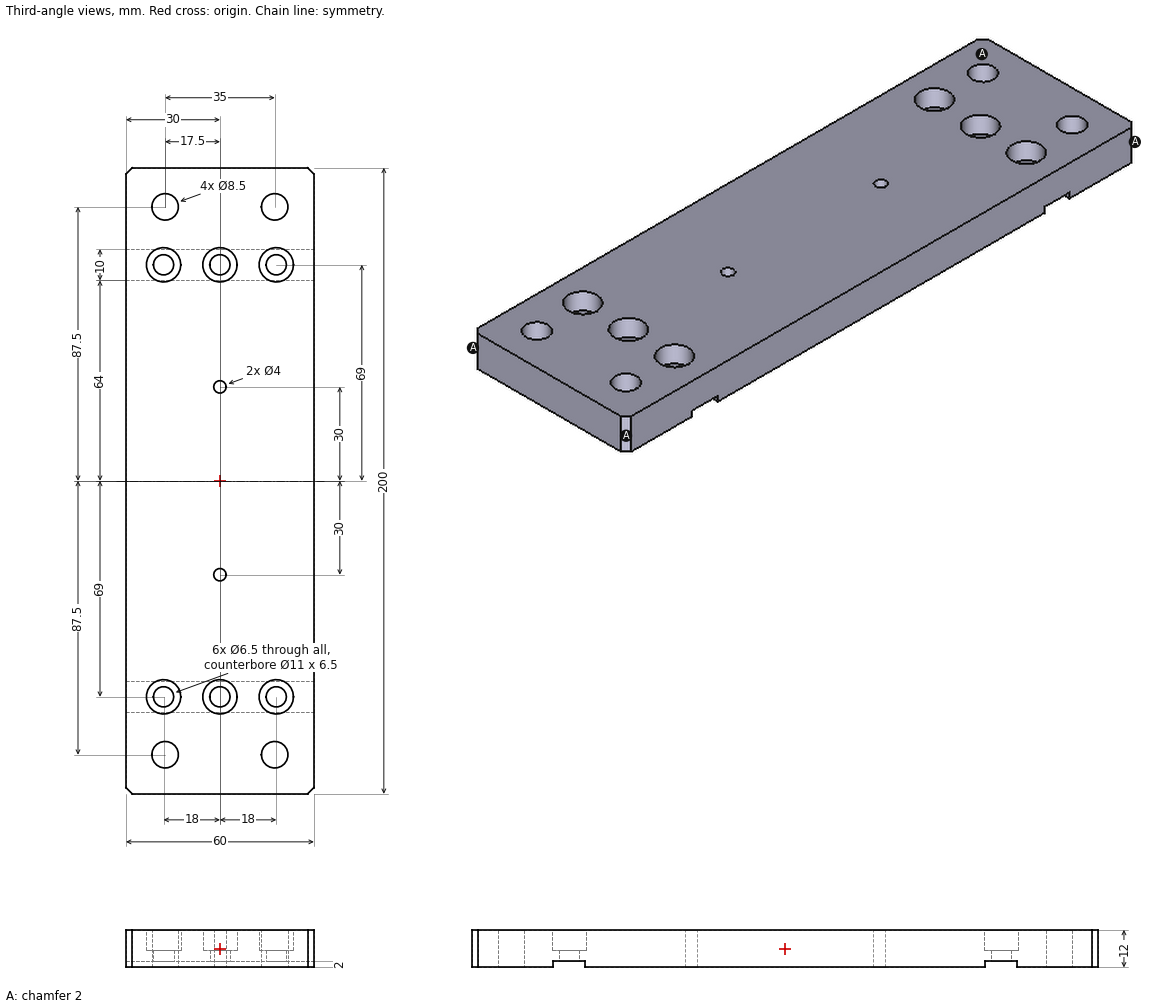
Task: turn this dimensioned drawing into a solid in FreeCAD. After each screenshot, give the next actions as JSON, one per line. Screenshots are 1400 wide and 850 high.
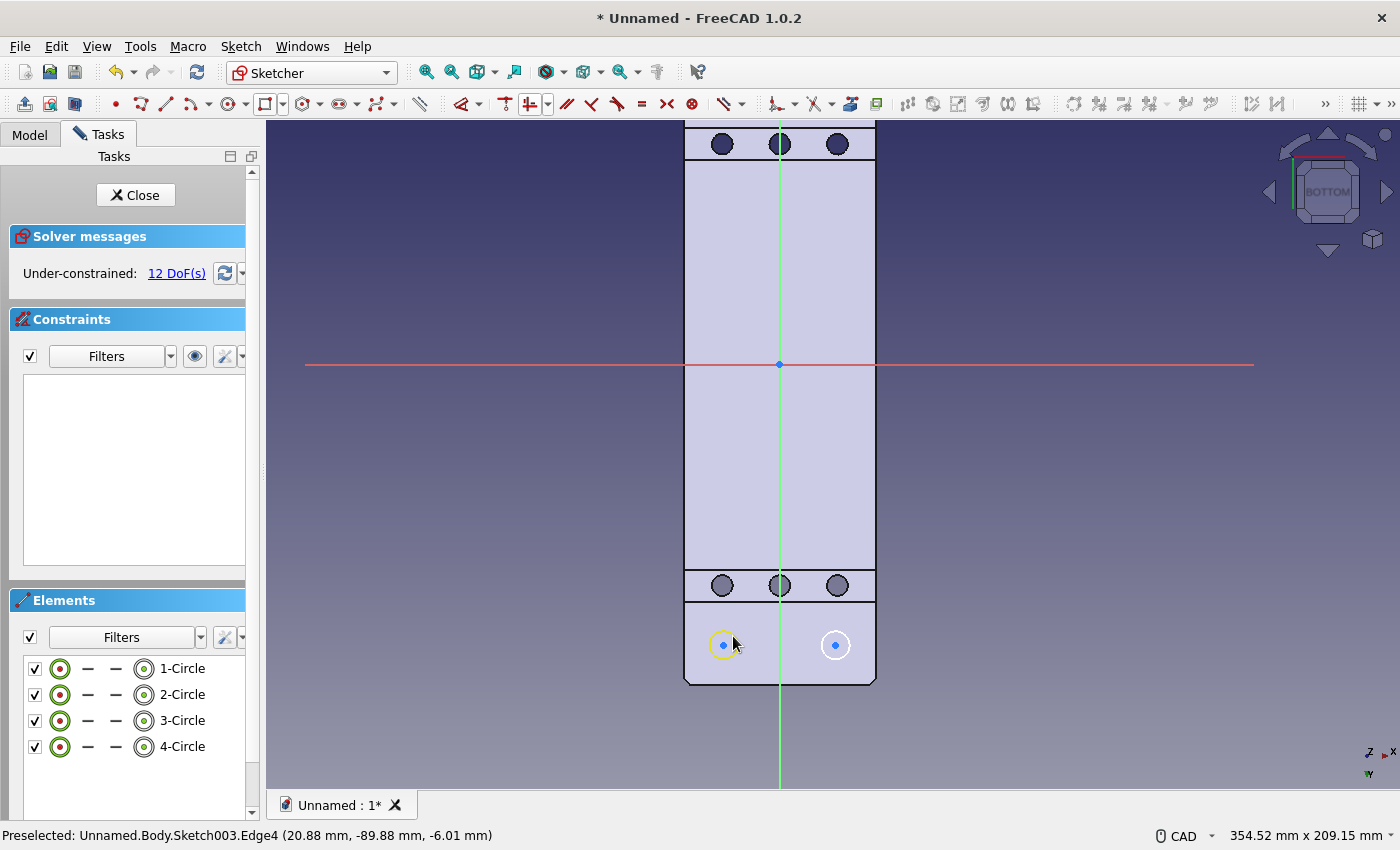
{"action": "left_click", "coordinate": [734, 635]}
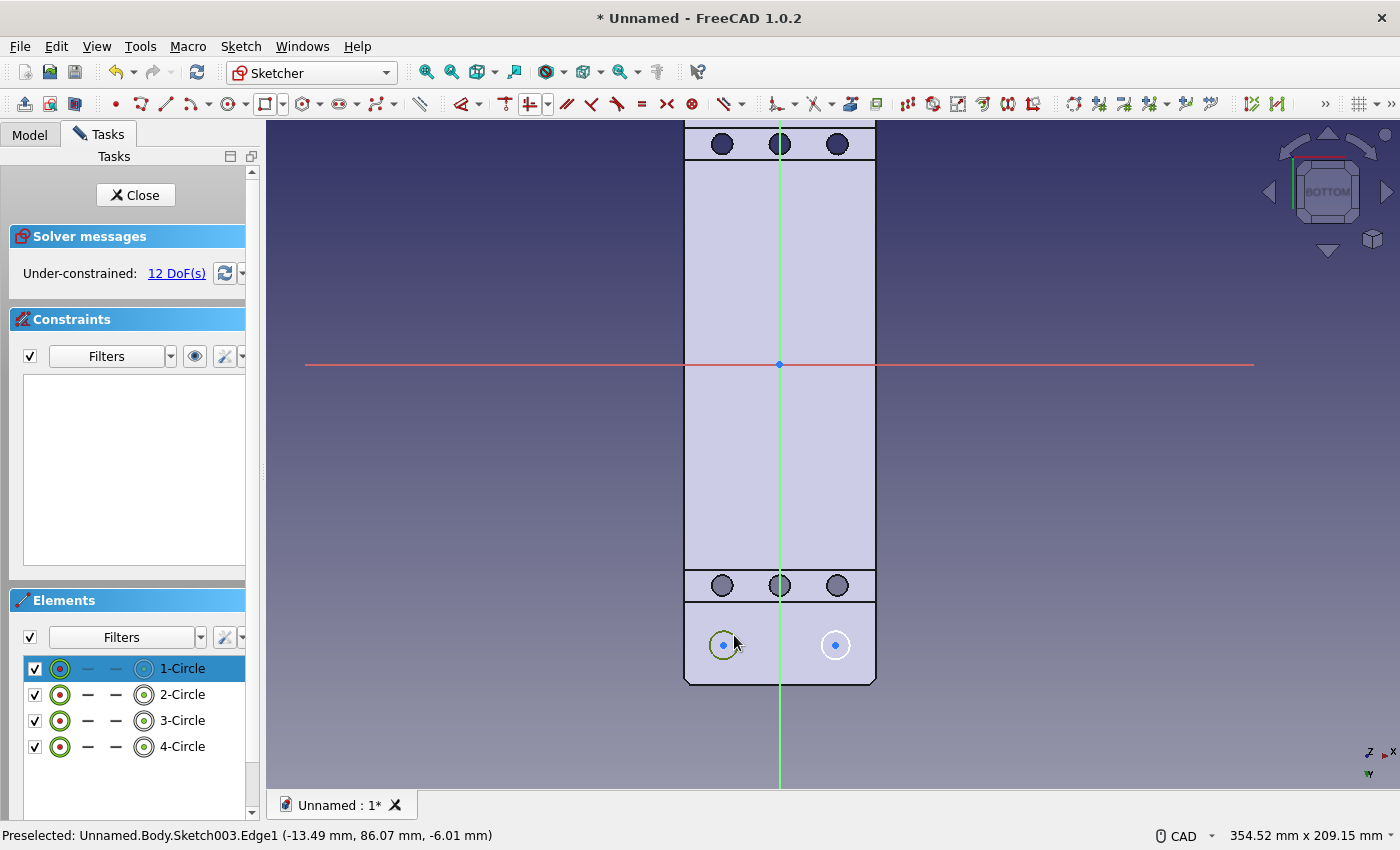
{"action": "left_click", "coordinate": [845, 635]}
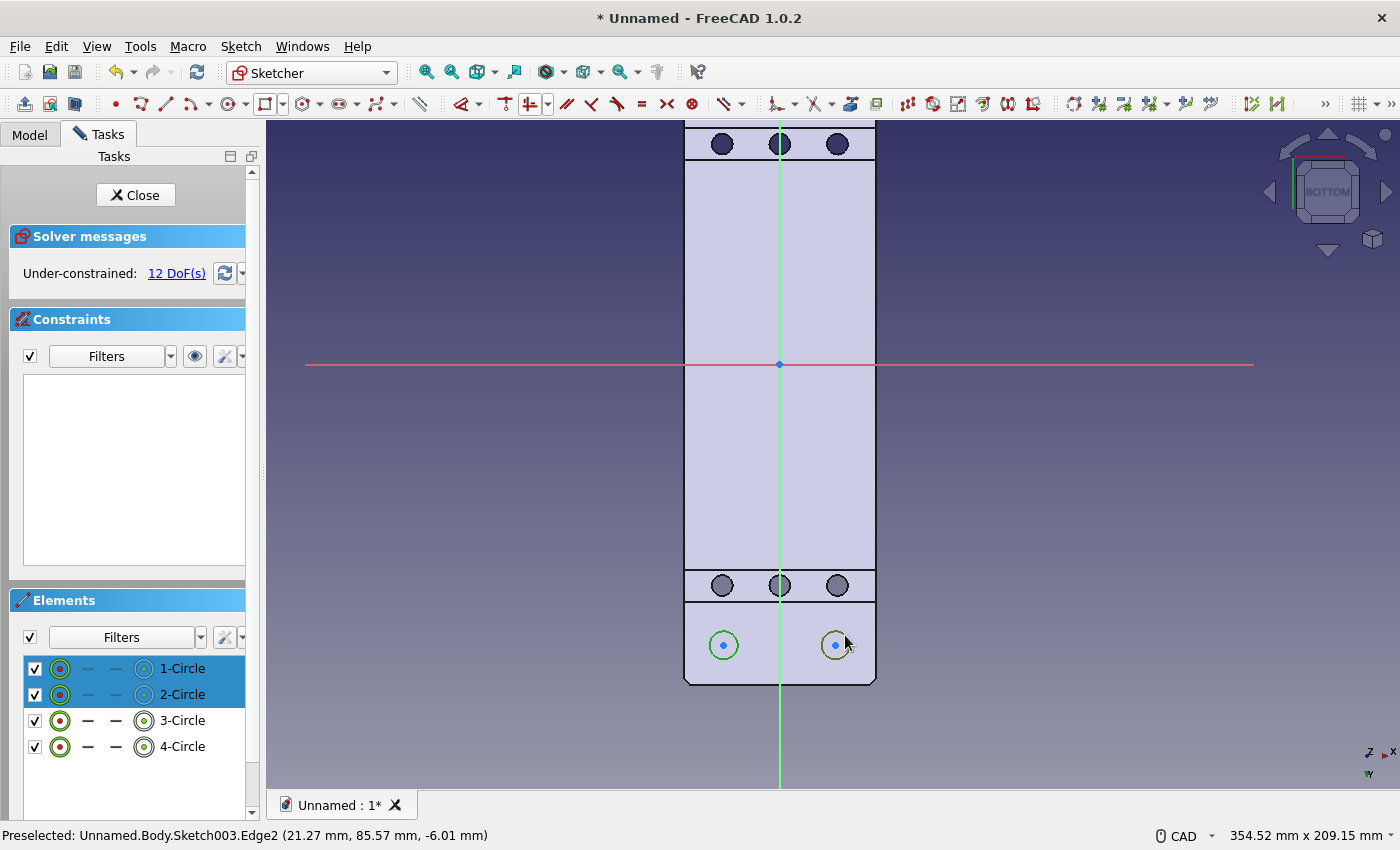
{"action": "scroll", "coordinate": [733, 637], "scroll_direction": "down", "scroll_amount": 2}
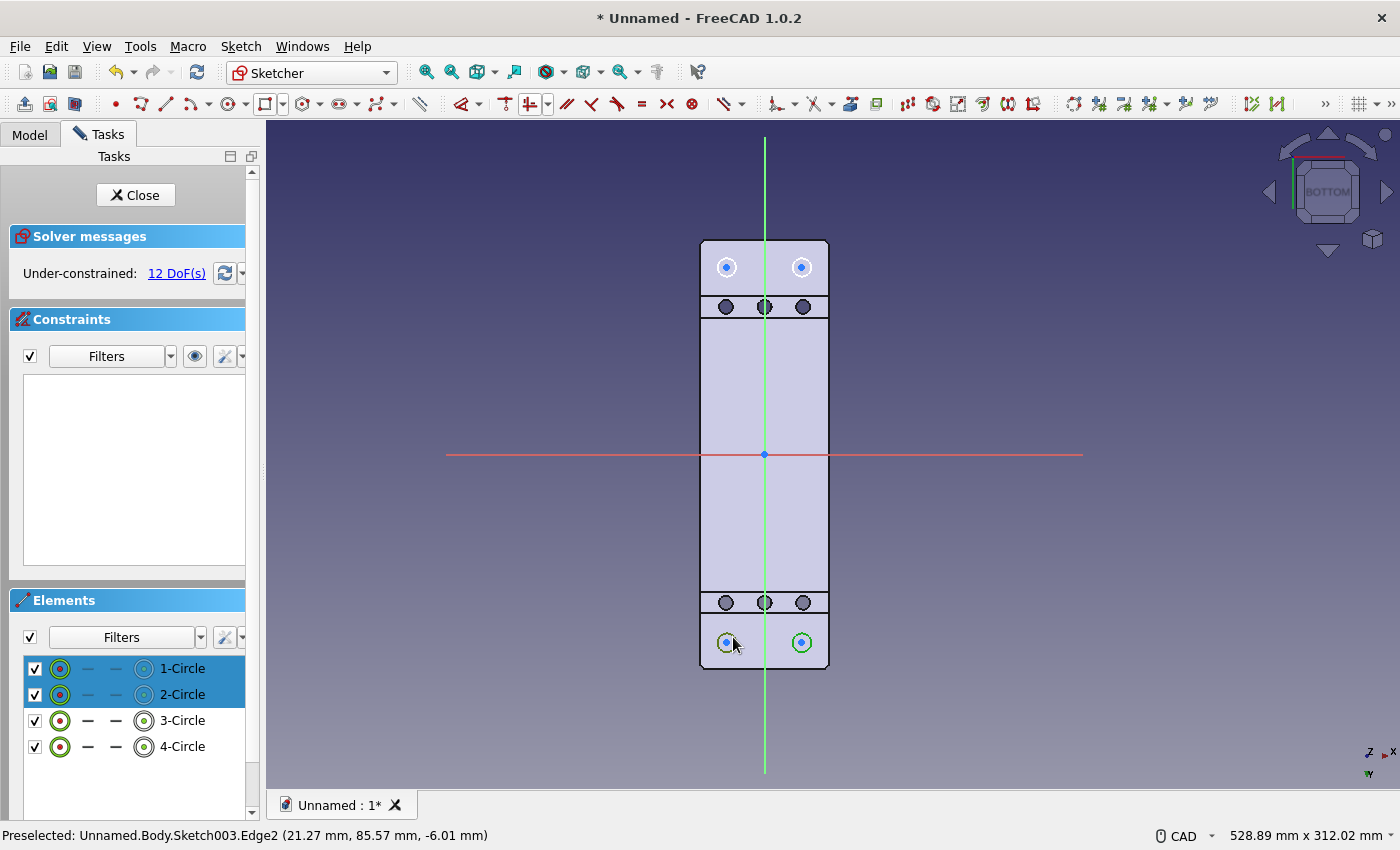
{"action": "scroll", "coordinate": [733, 261], "scroll_direction": "up", "scroll_amount": 3}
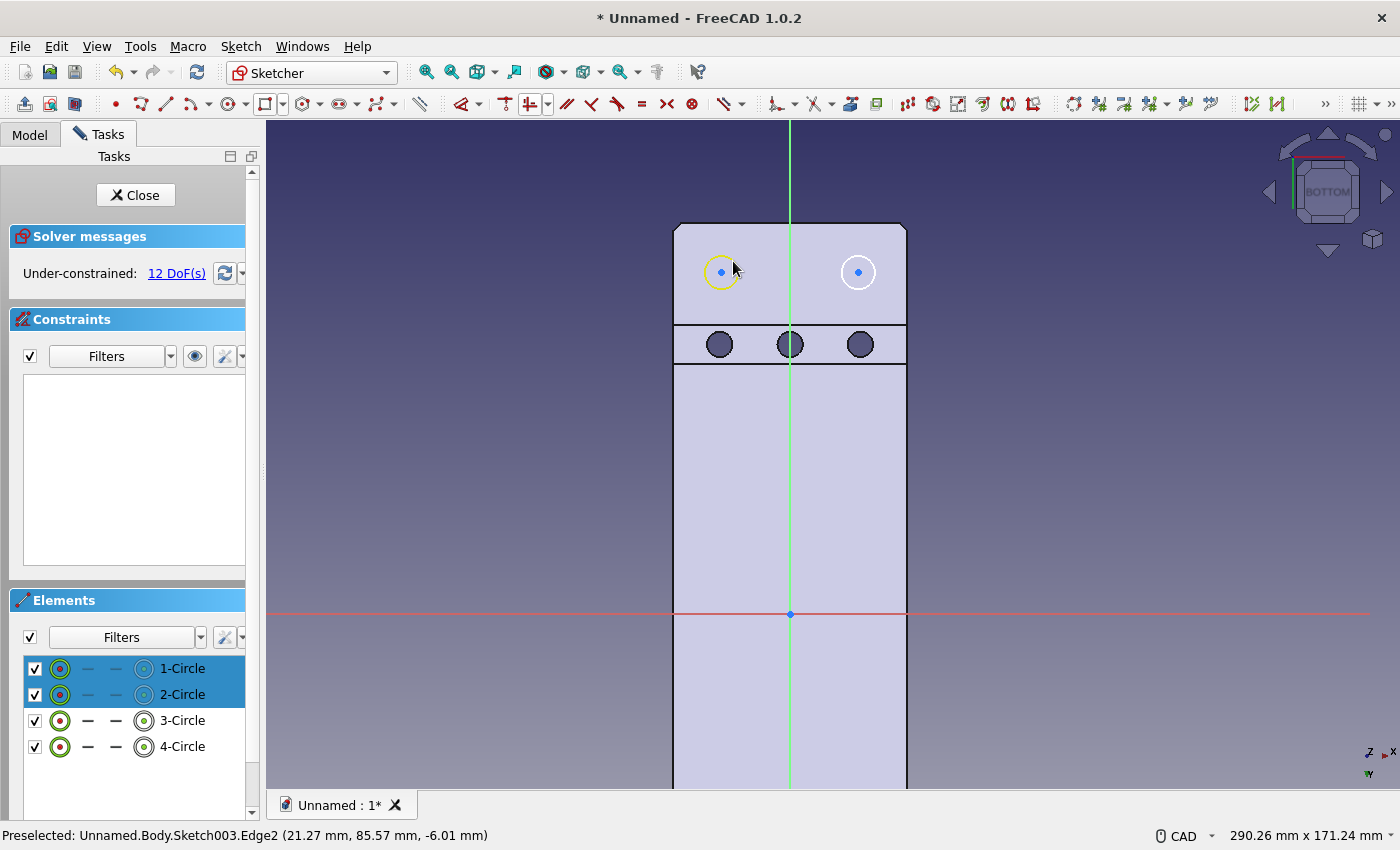
{"action": "left_click", "coordinate": [733, 261]}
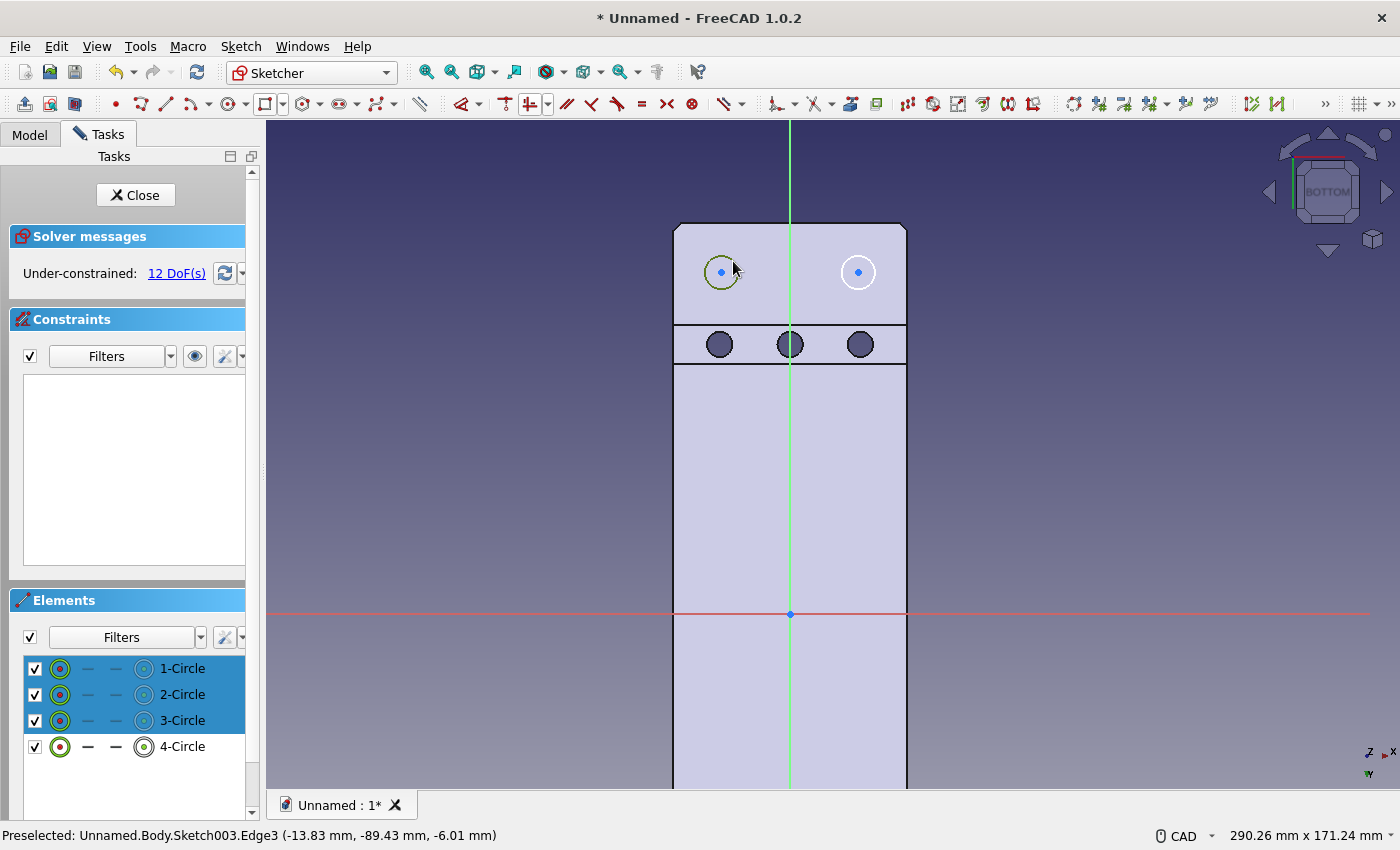
{"action": "left_click", "coordinate": [870, 261]}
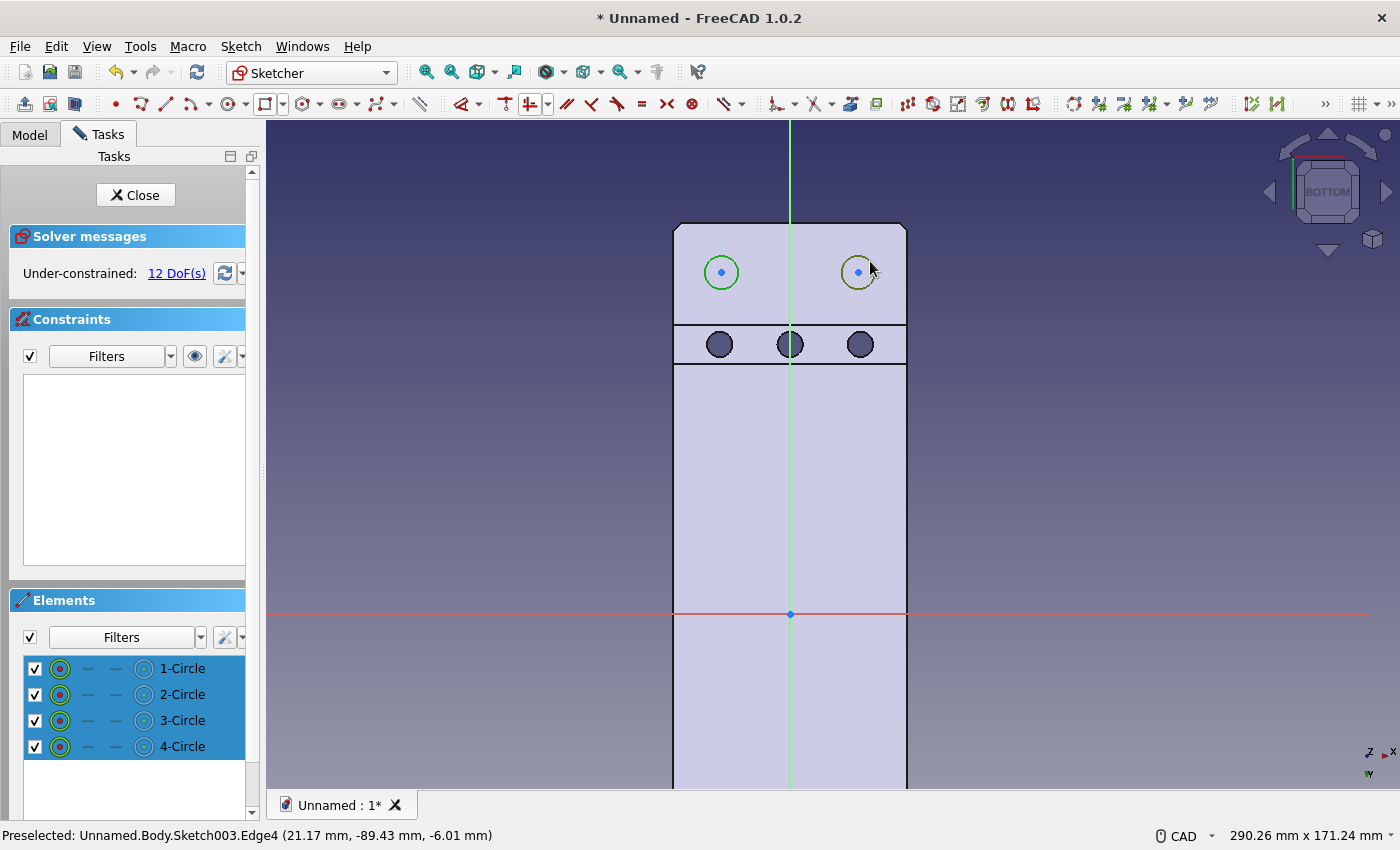
{"action": "left_click", "coordinate": [642, 104]}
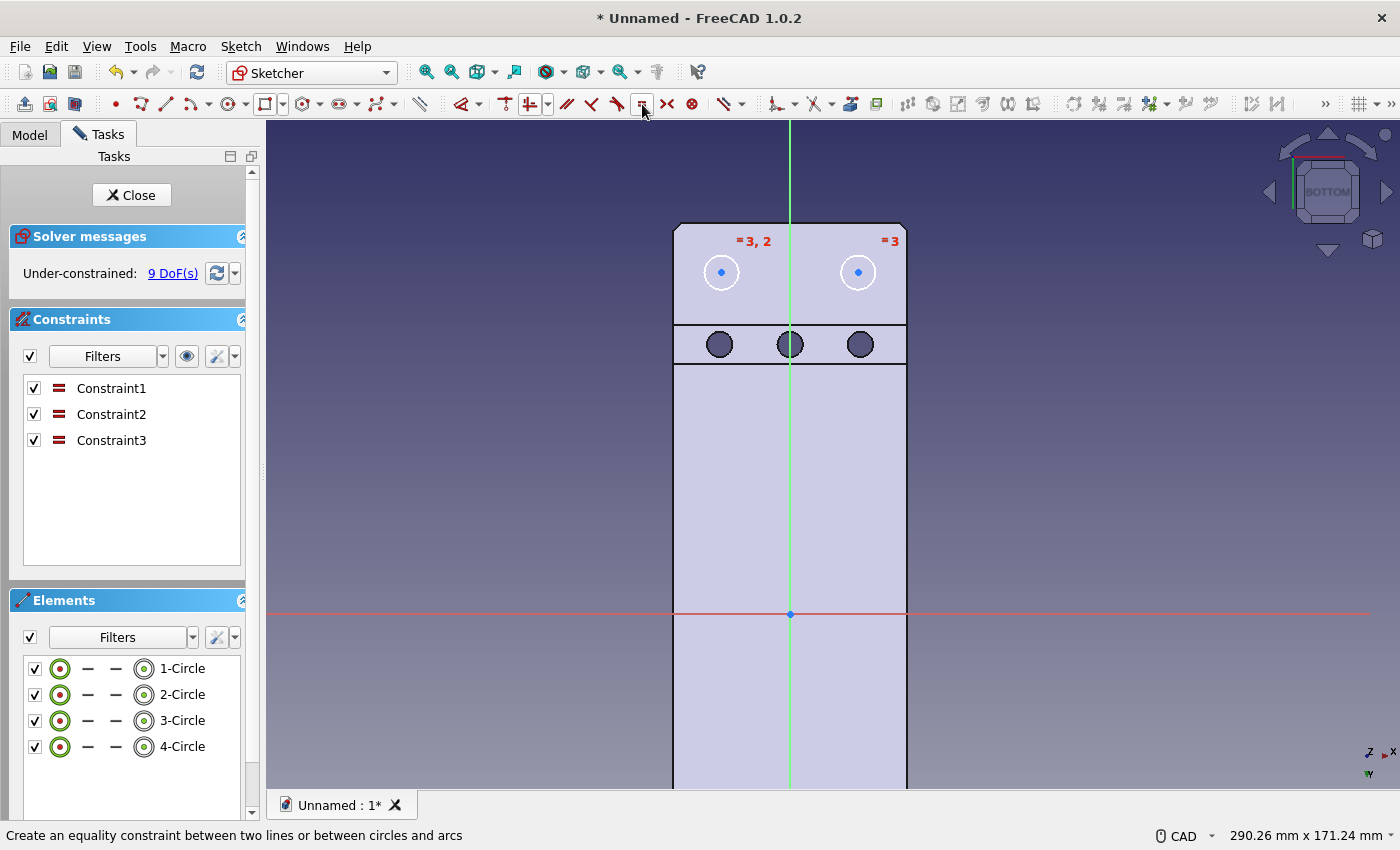
{"action": "scroll", "coordinate": [733, 260], "scroll_direction": "down", "scroll_amount": 3}